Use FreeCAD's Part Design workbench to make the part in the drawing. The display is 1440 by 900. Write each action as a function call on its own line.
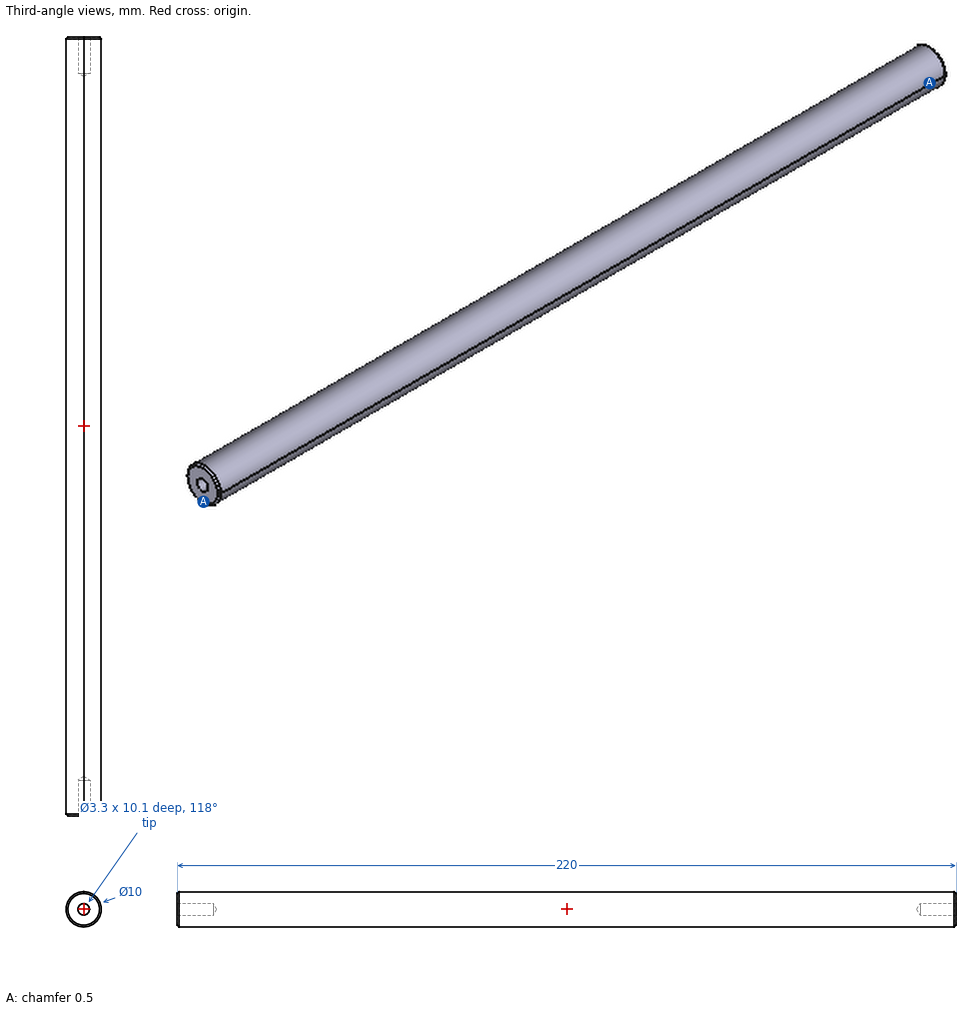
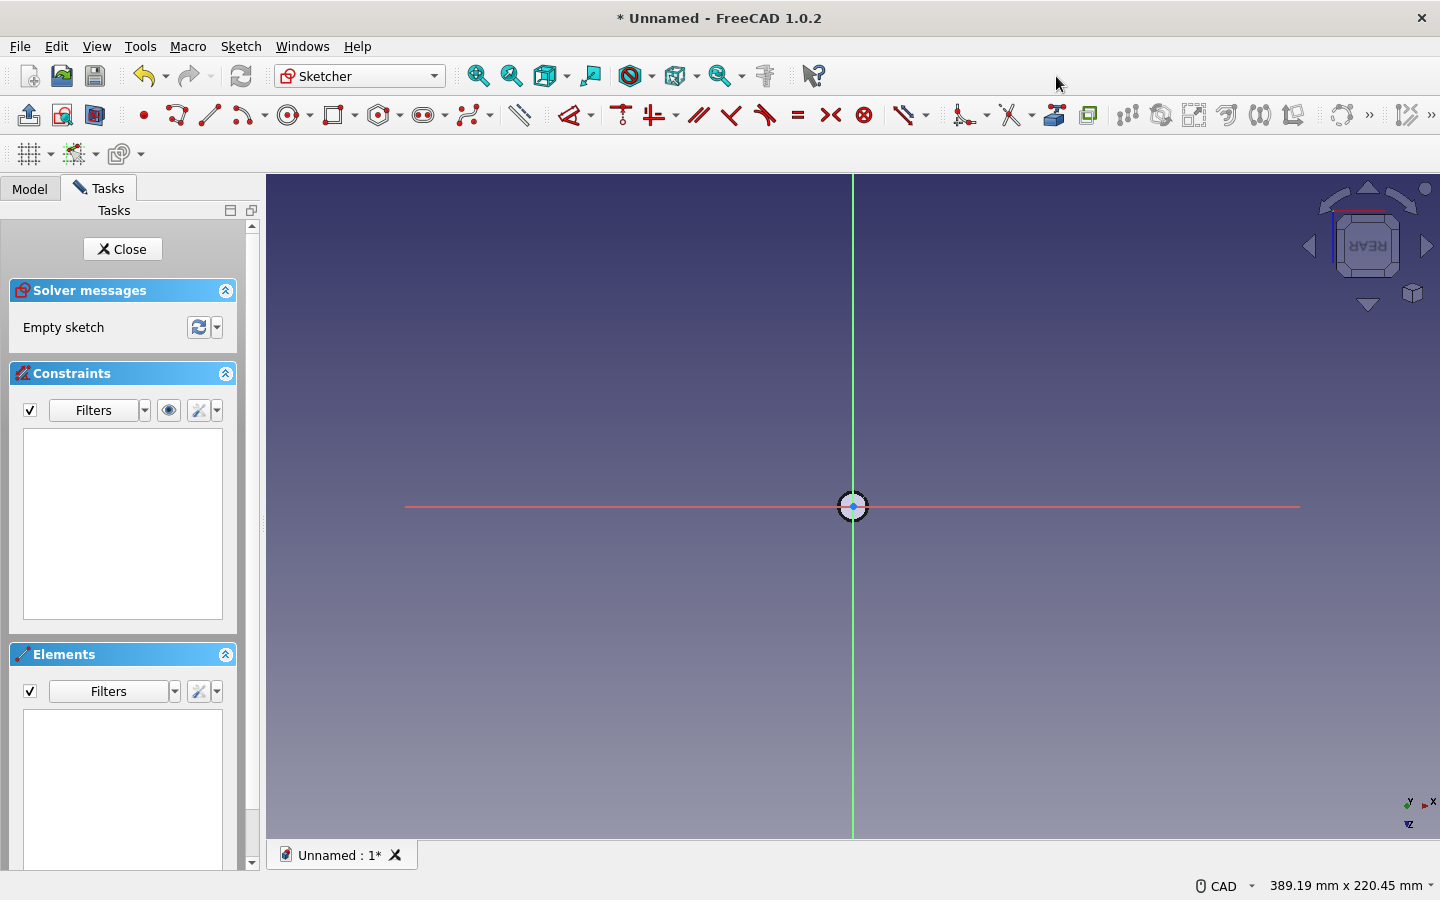
scroll(857, 506, up, 15)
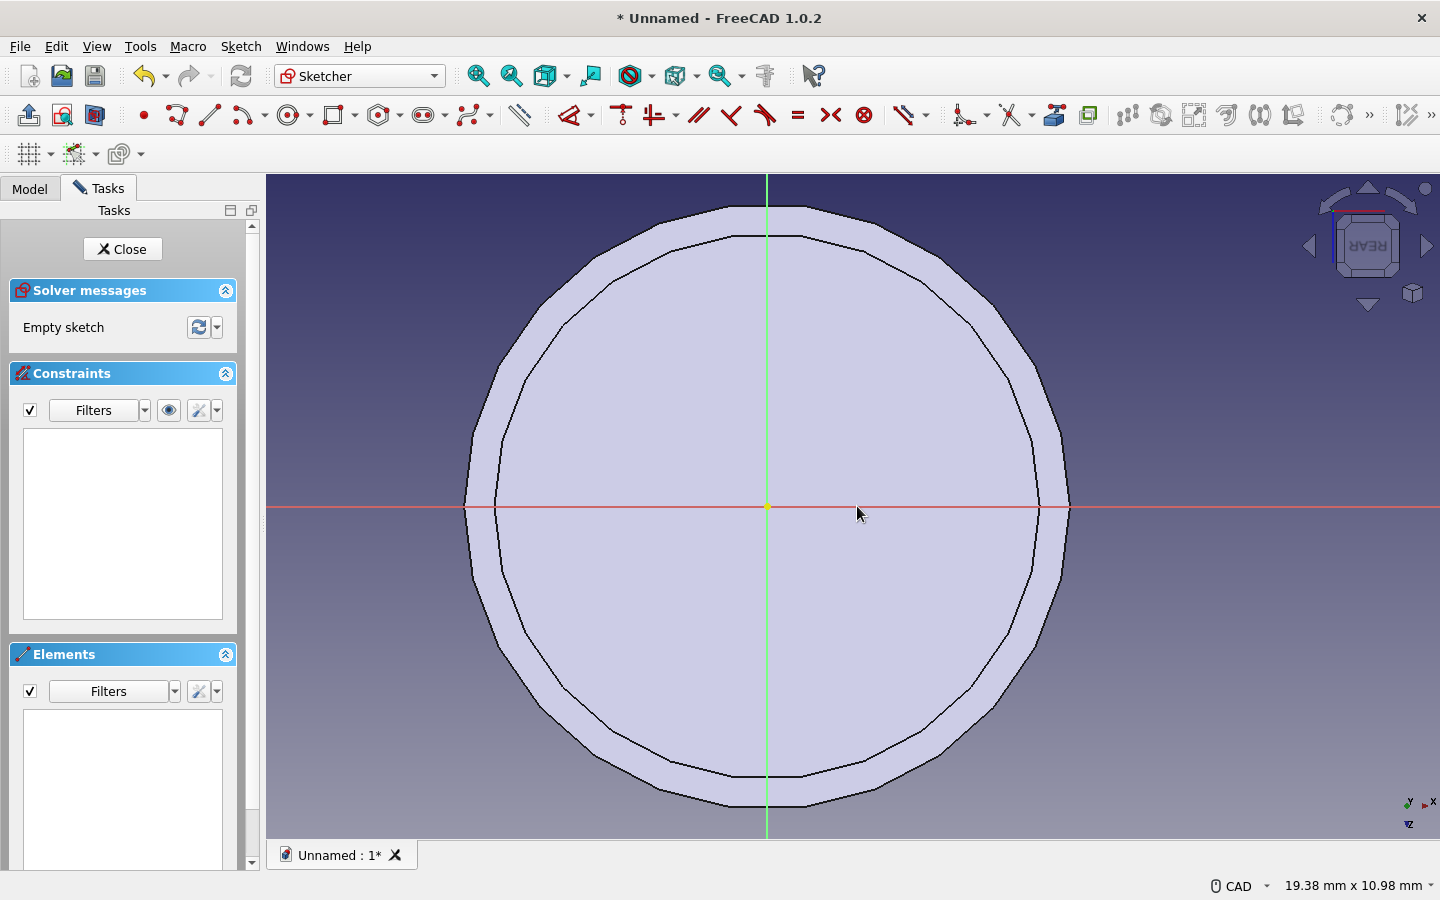
scroll(753, 506, up, 4)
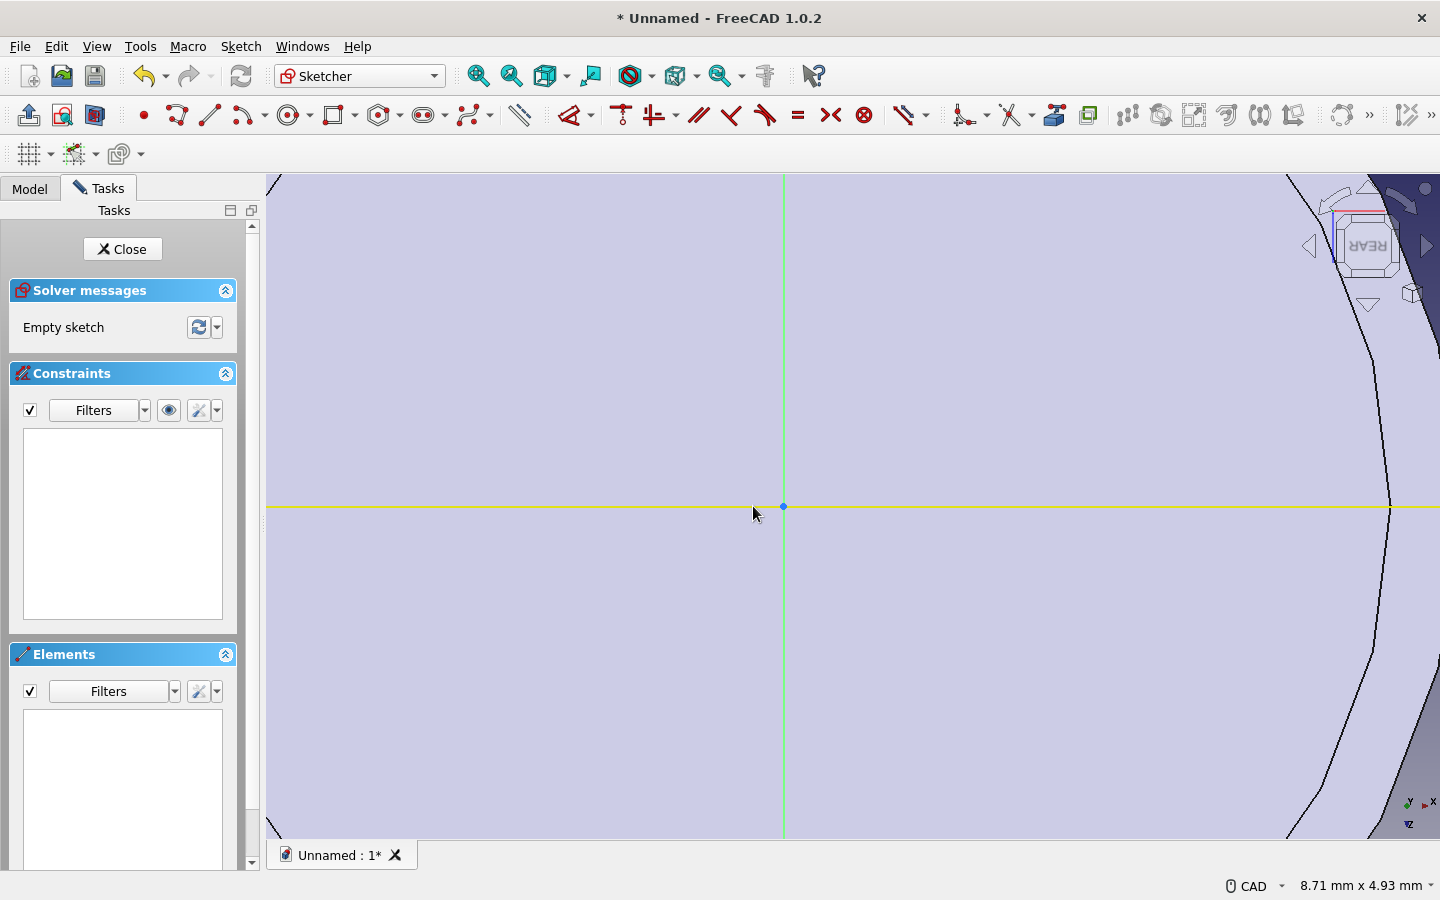
key(g)
key(c)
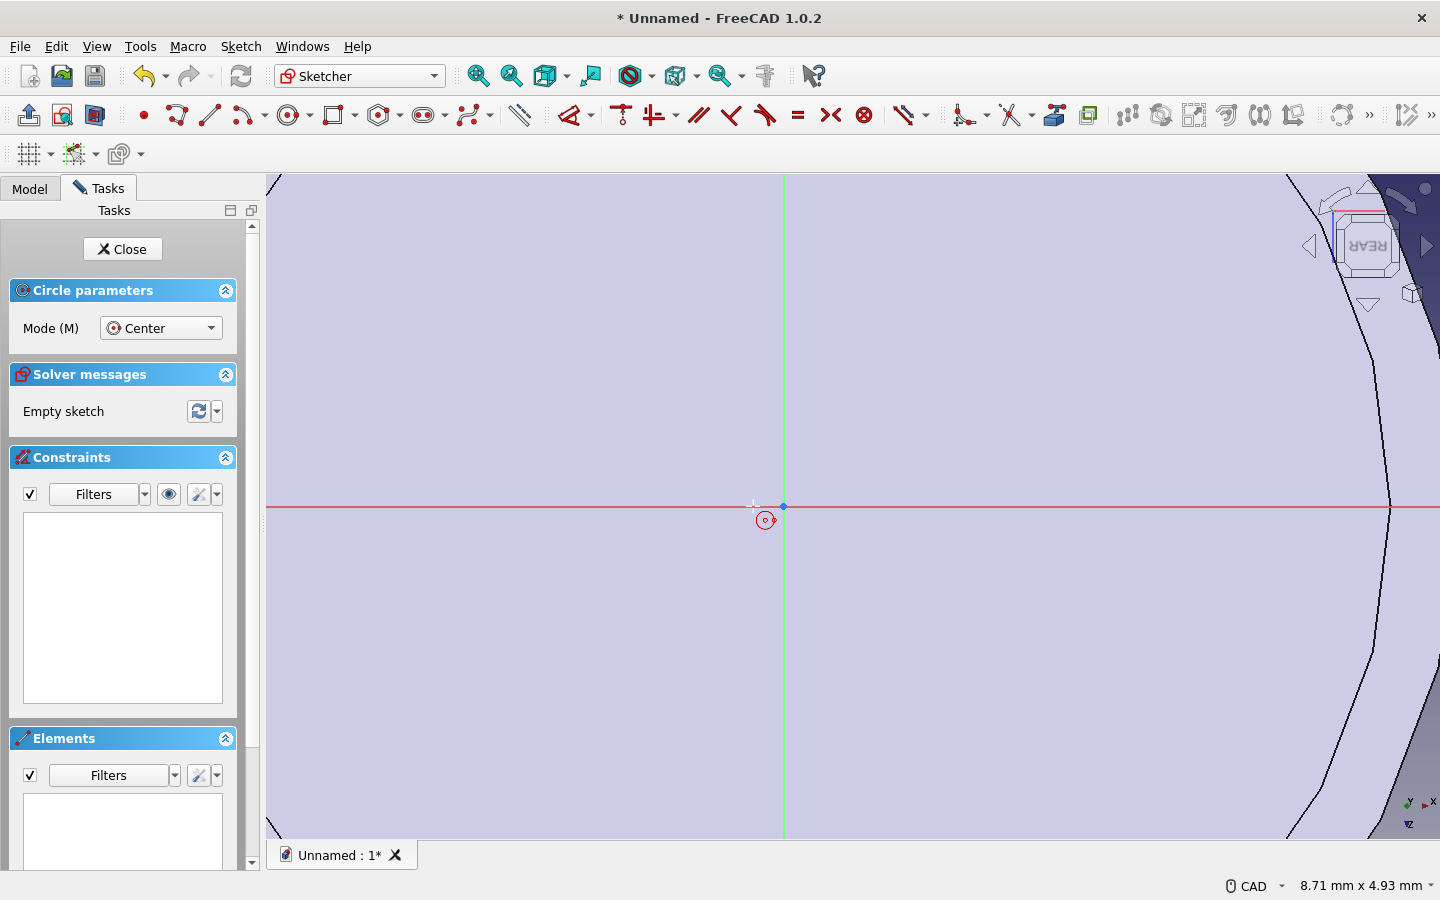
click(784, 506)
move(941, 349)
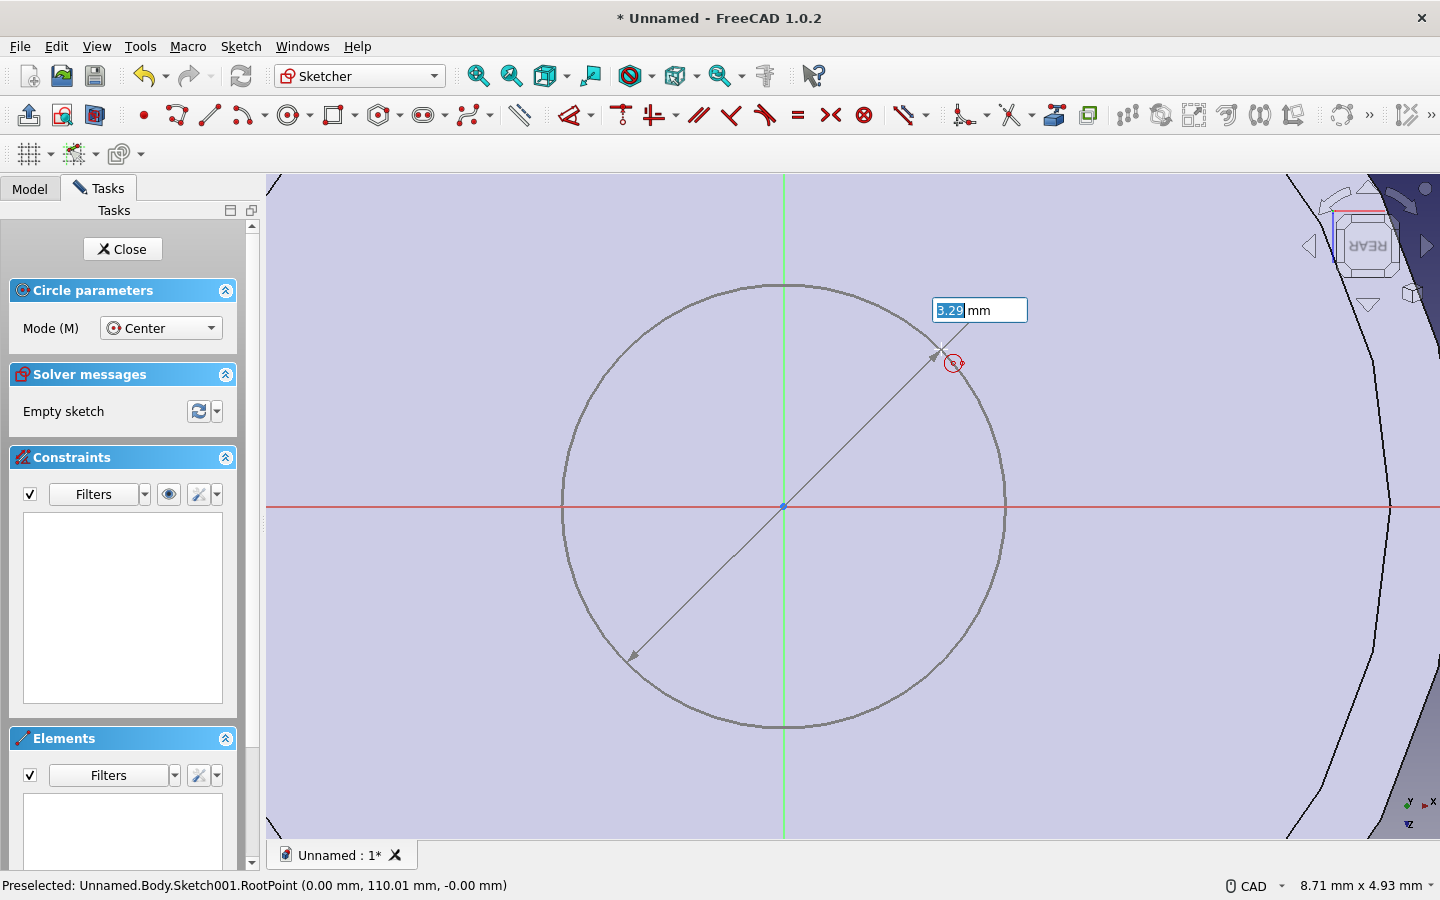
text(3.3)
key(Return)
key(Escape)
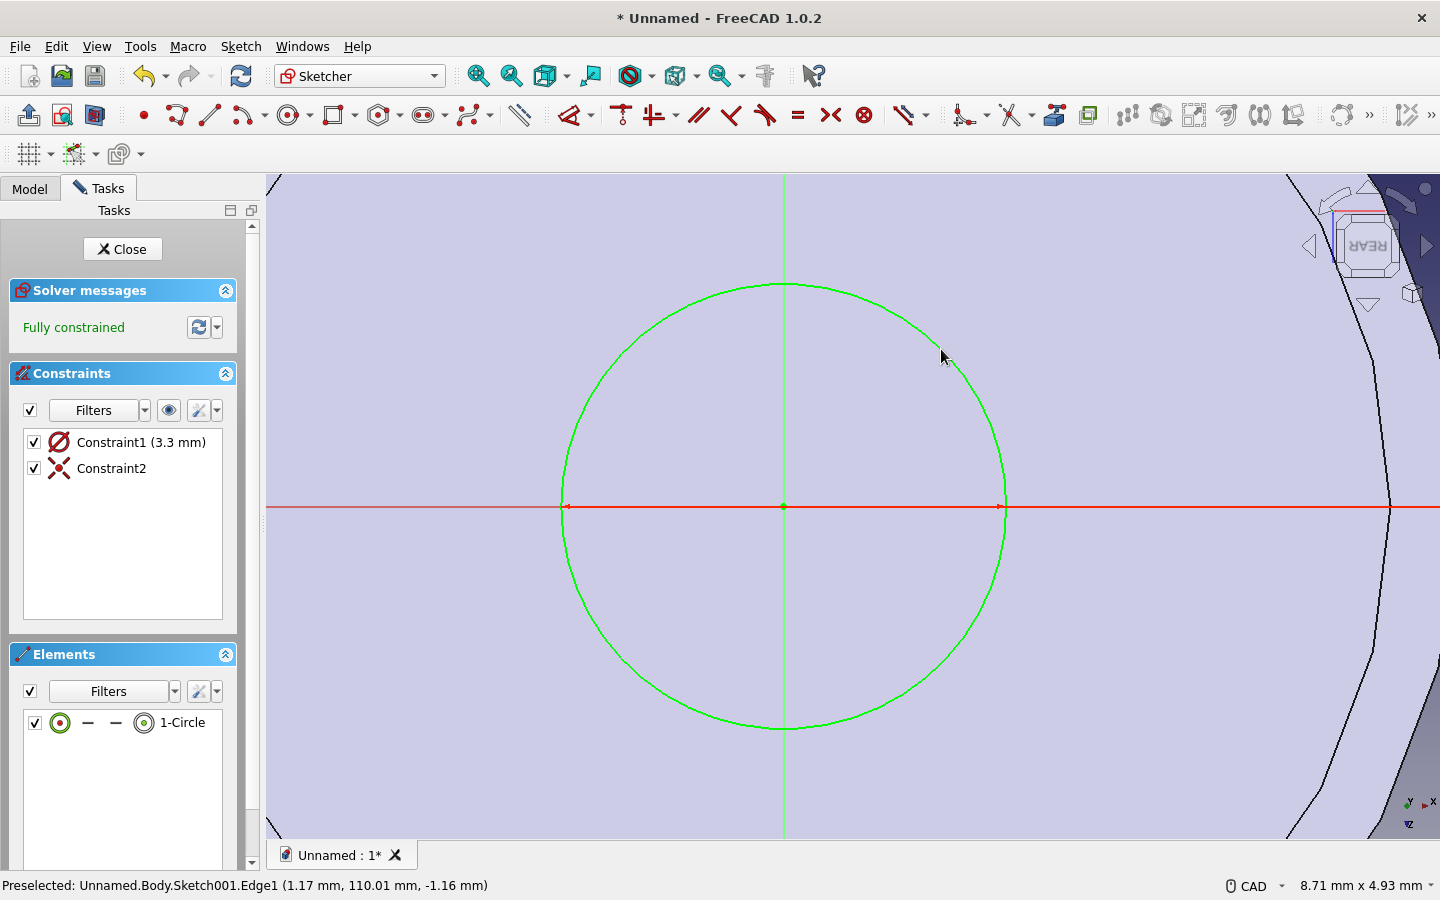
click(123, 249)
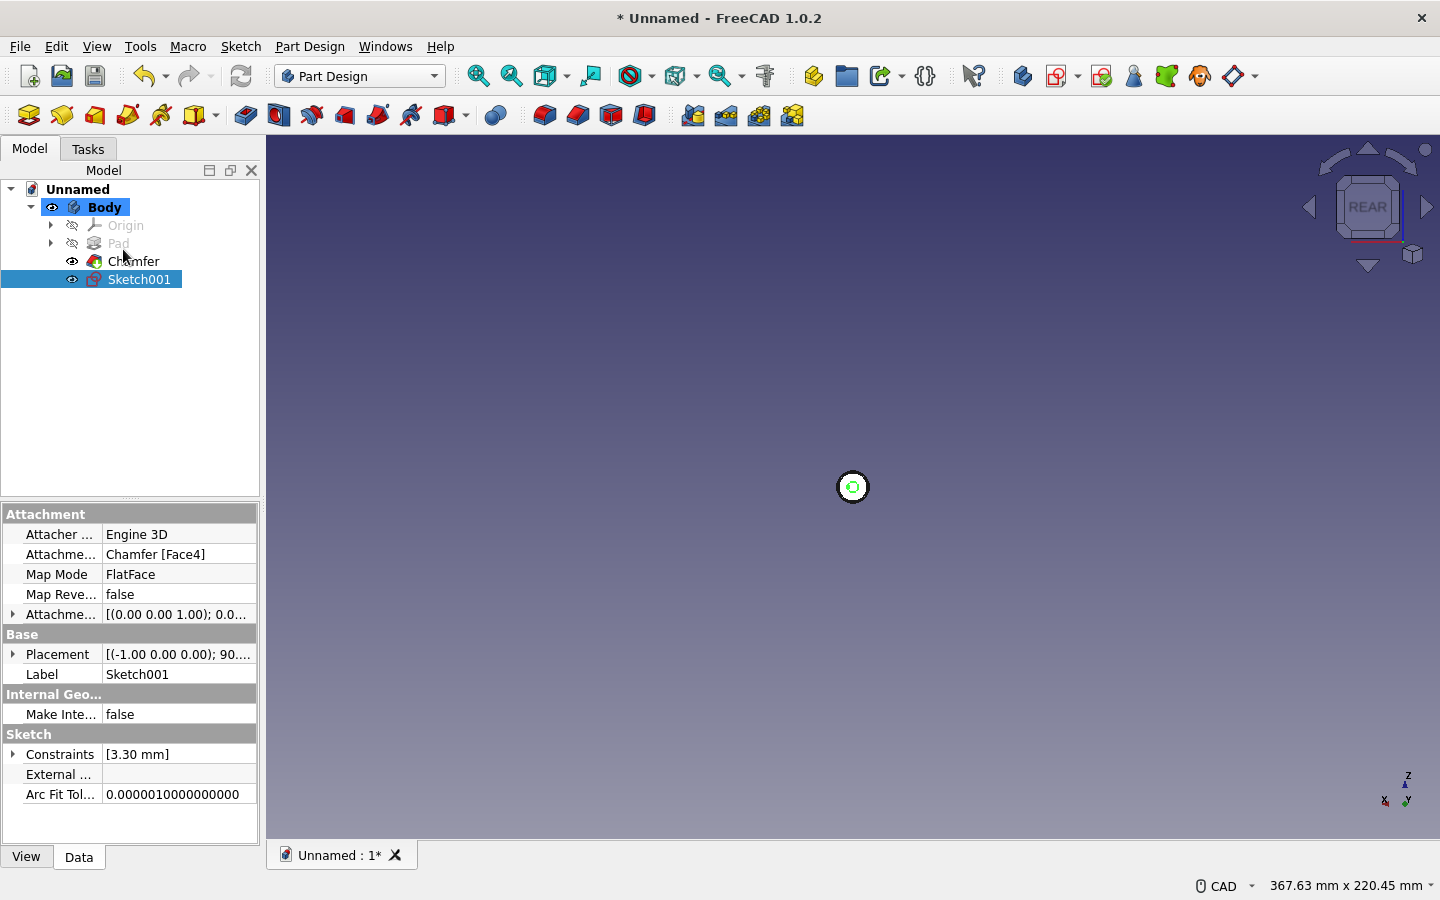
click(279, 116)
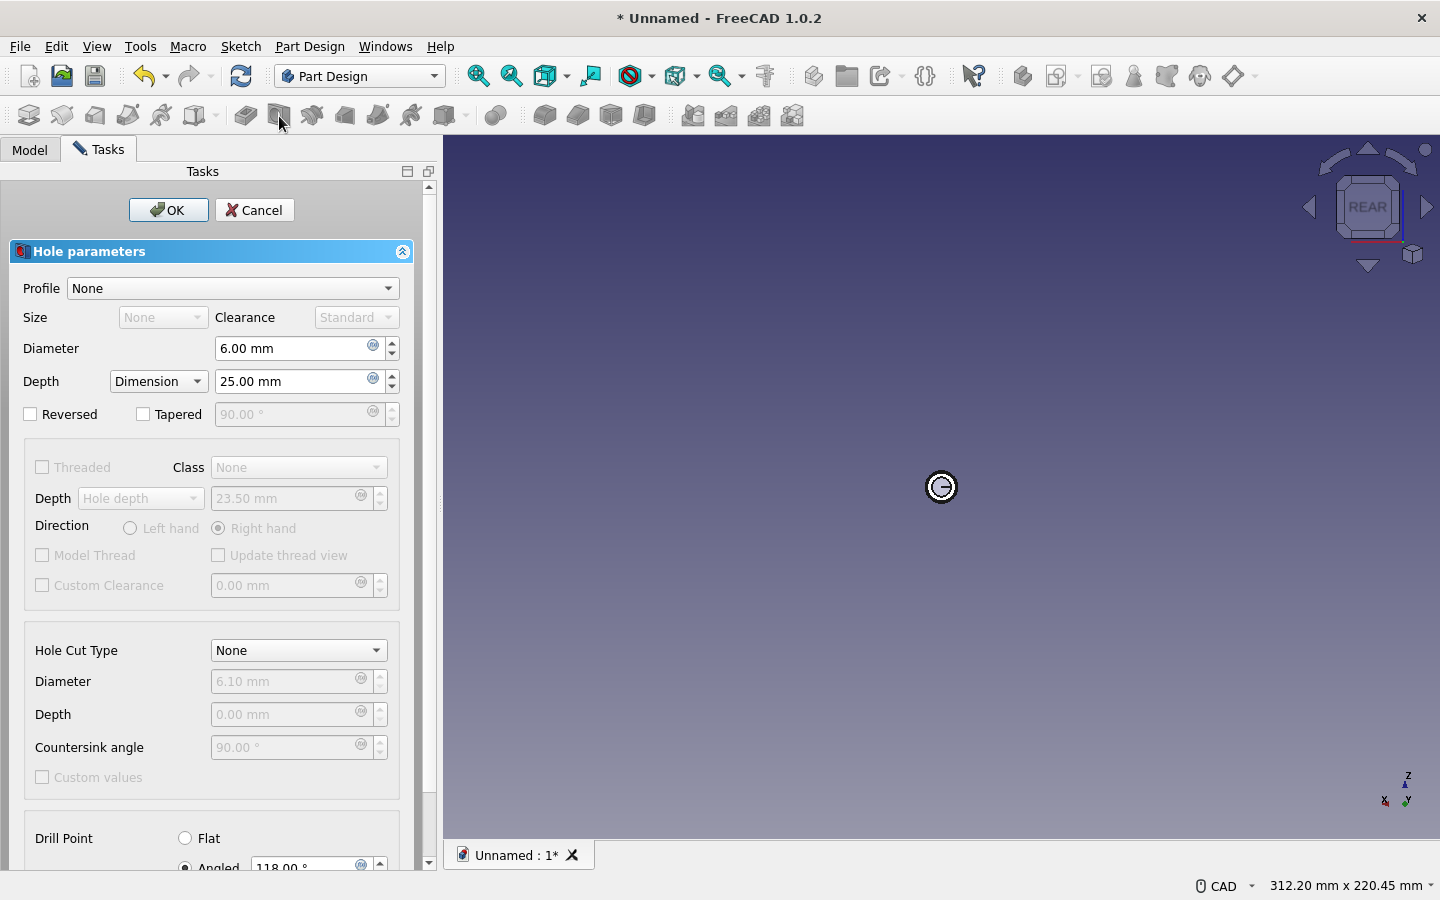
triple_click(300, 348)